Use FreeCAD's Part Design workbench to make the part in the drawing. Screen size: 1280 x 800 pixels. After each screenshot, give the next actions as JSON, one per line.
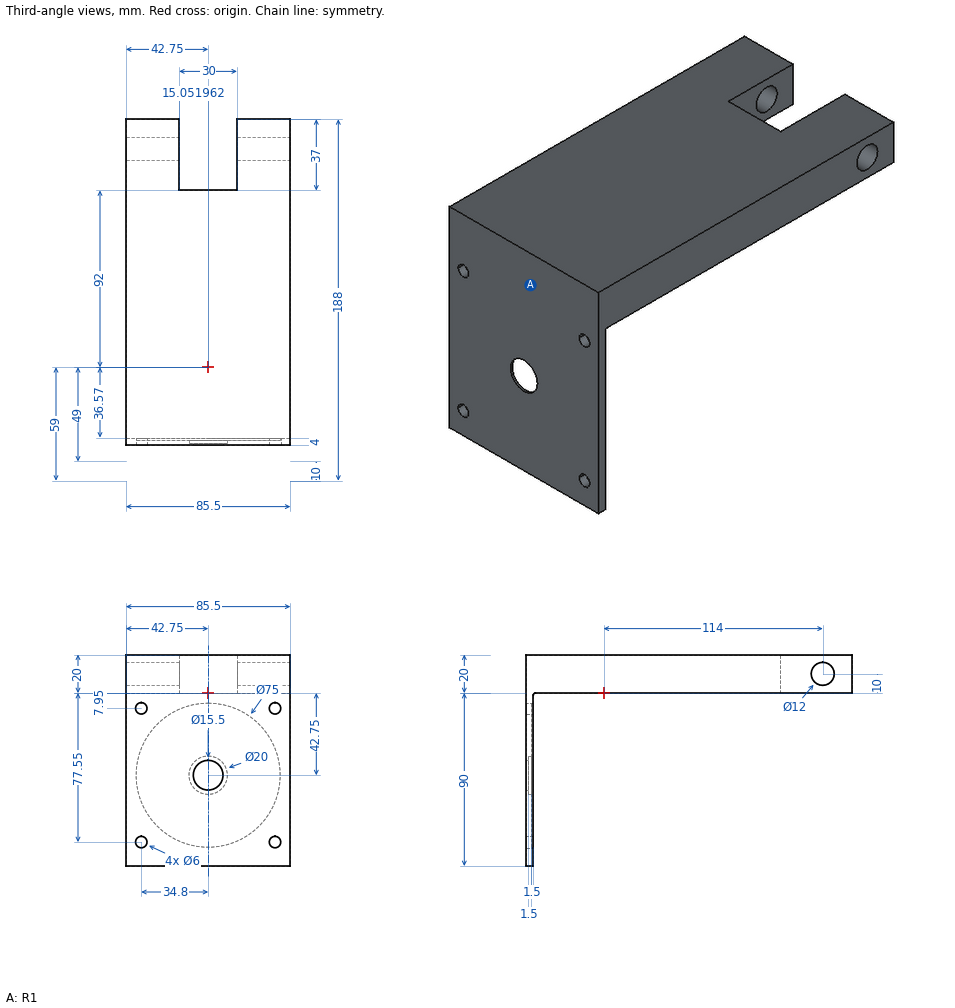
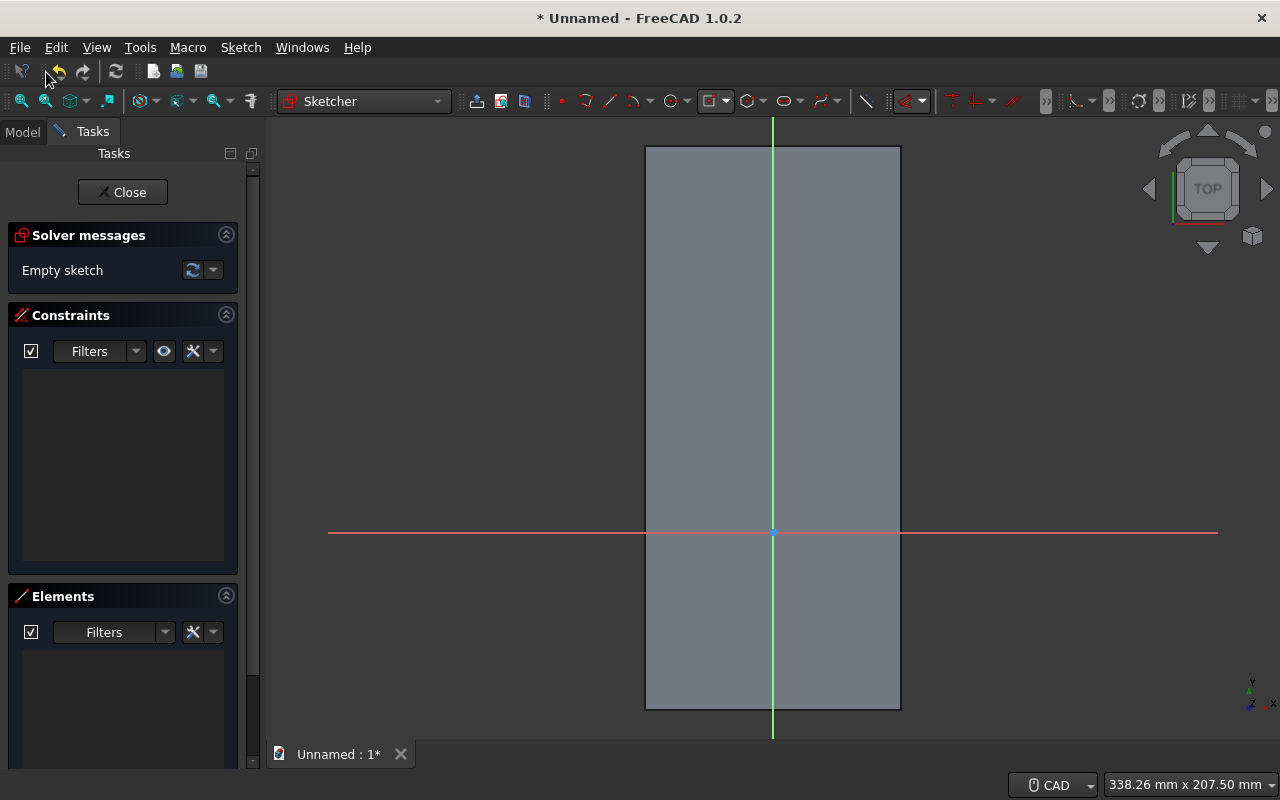
{"action": "scroll", "coordinate": [704, 428], "scroll_direction": "down", "scroll_amount": 5}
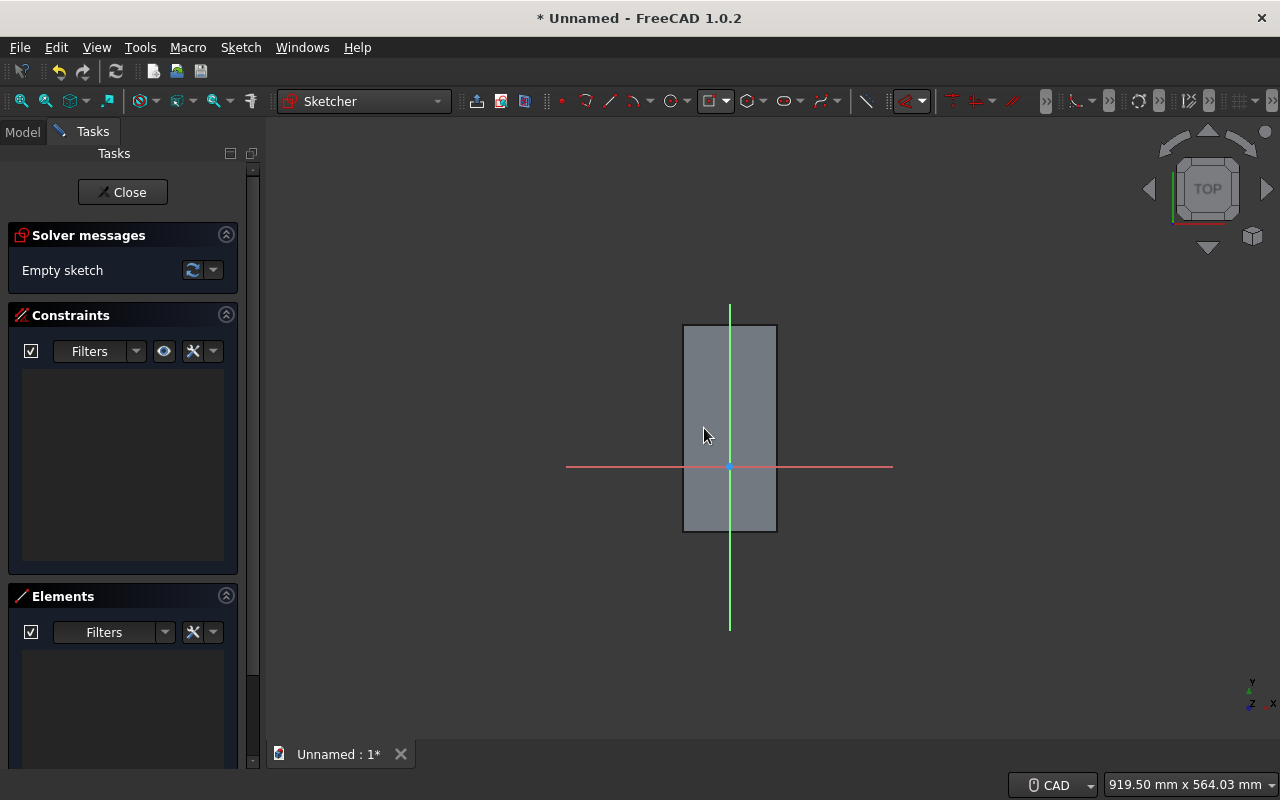
{"action": "scroll", "coordinate": [733, 335], "scroll_direction": "up", "scroll_amount": 11}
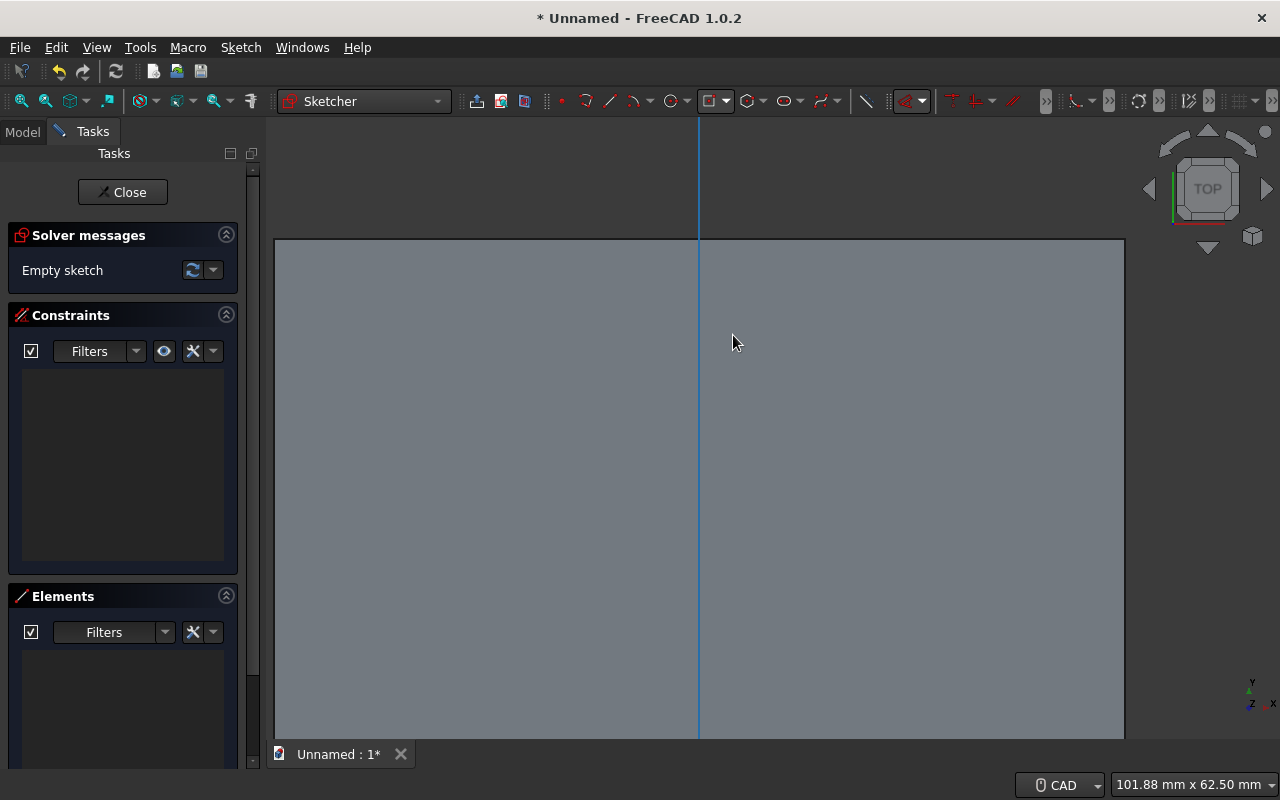
{"action": "key", "text": "g r"}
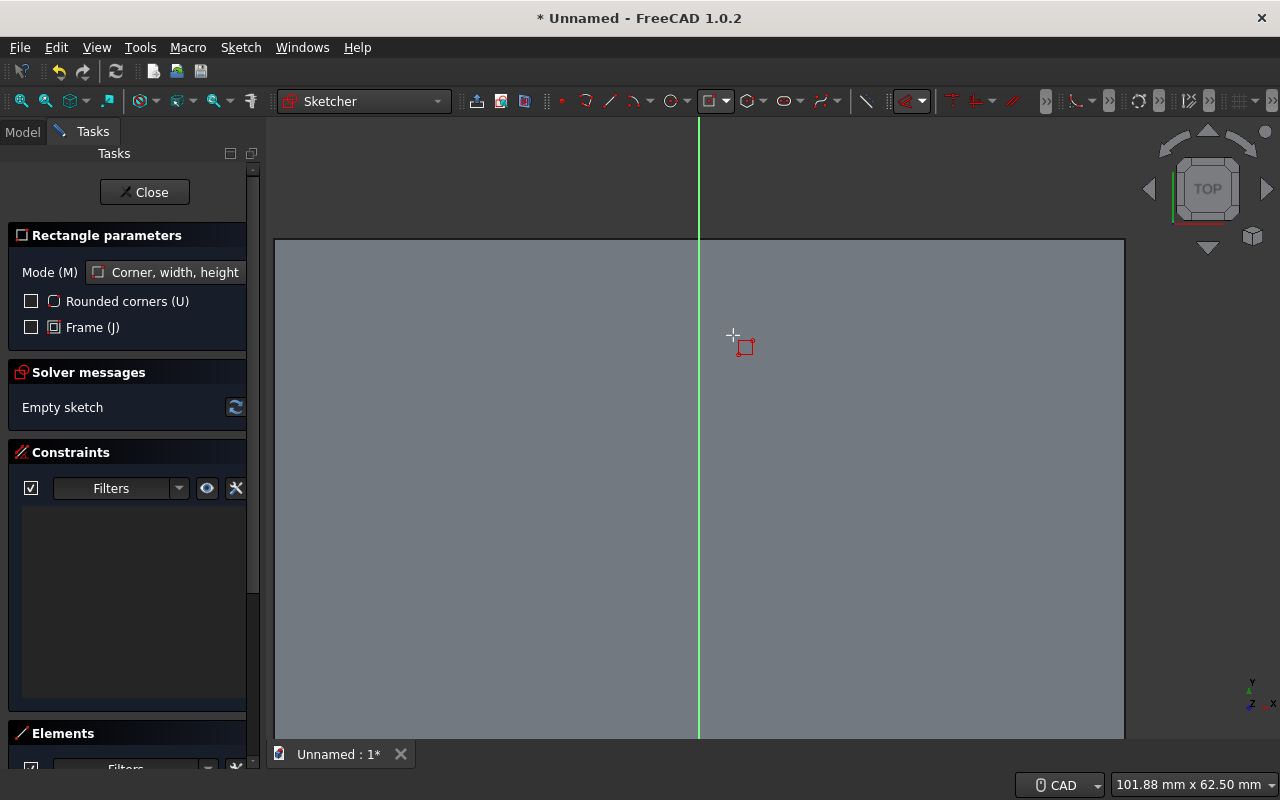
{"action": "left_click", "coordinate": [549, 239]}
{"action": "mouse_move", "coordinate": [848, 607]}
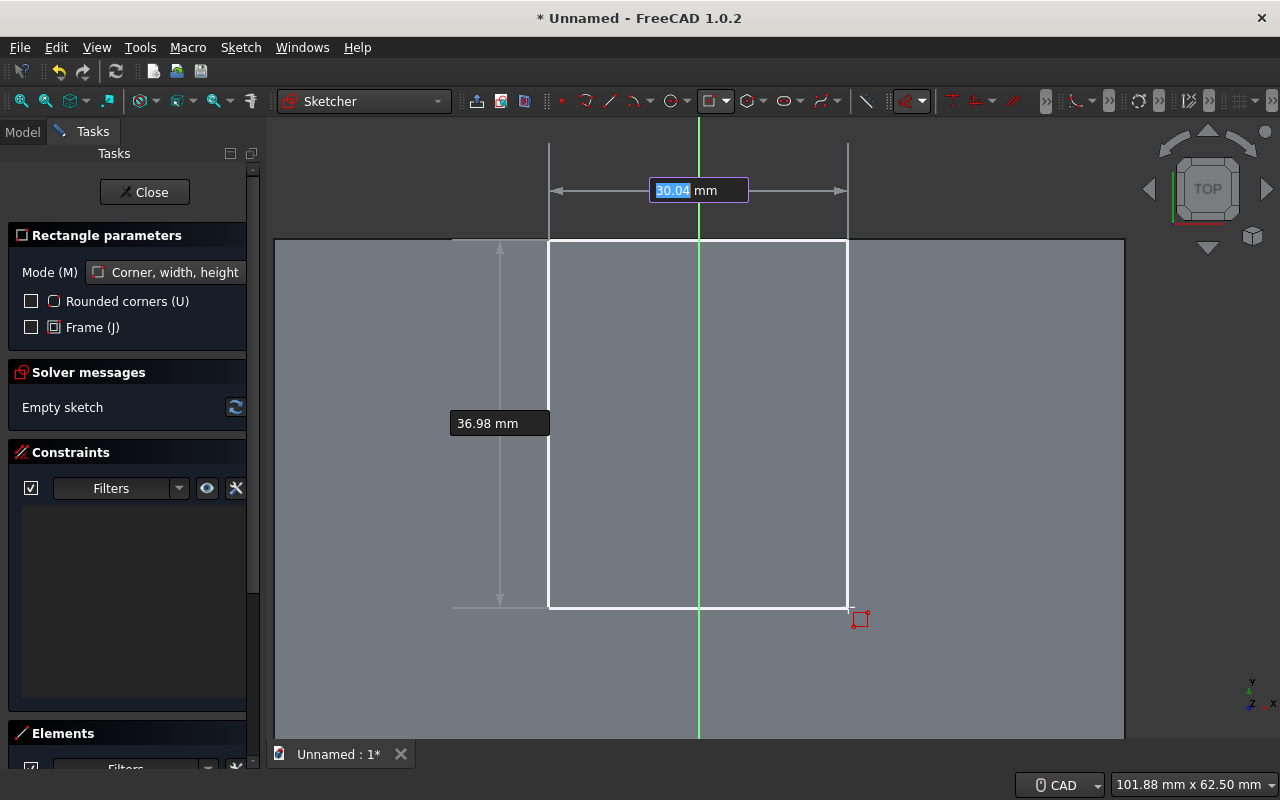
{"action": "type", "text": "30"}
{"action": "key", "text": "Tab"}
{"action": "type", "text": "37"}
{"action": "key", "text": "Return"}
{"action": "key", "text": "Escape"}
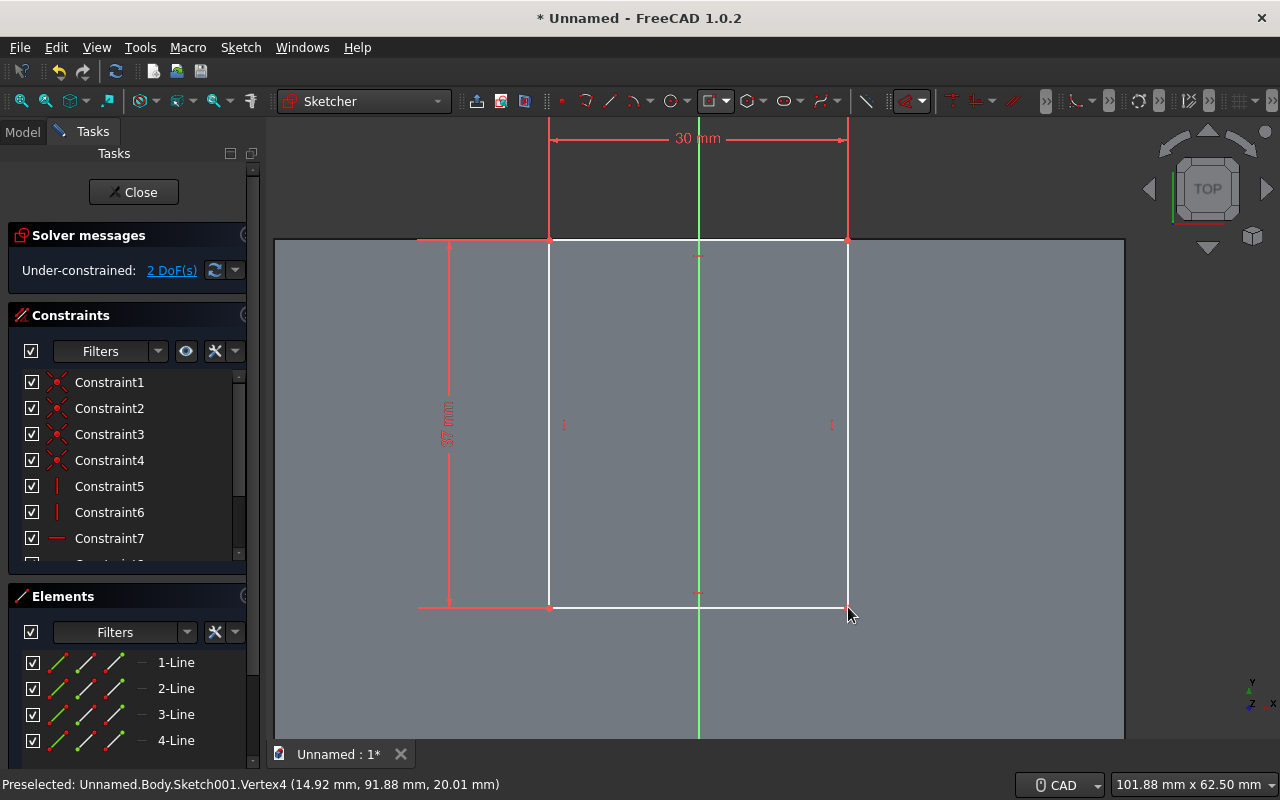
{"action": "left_click", "coordinate": [906, 102]}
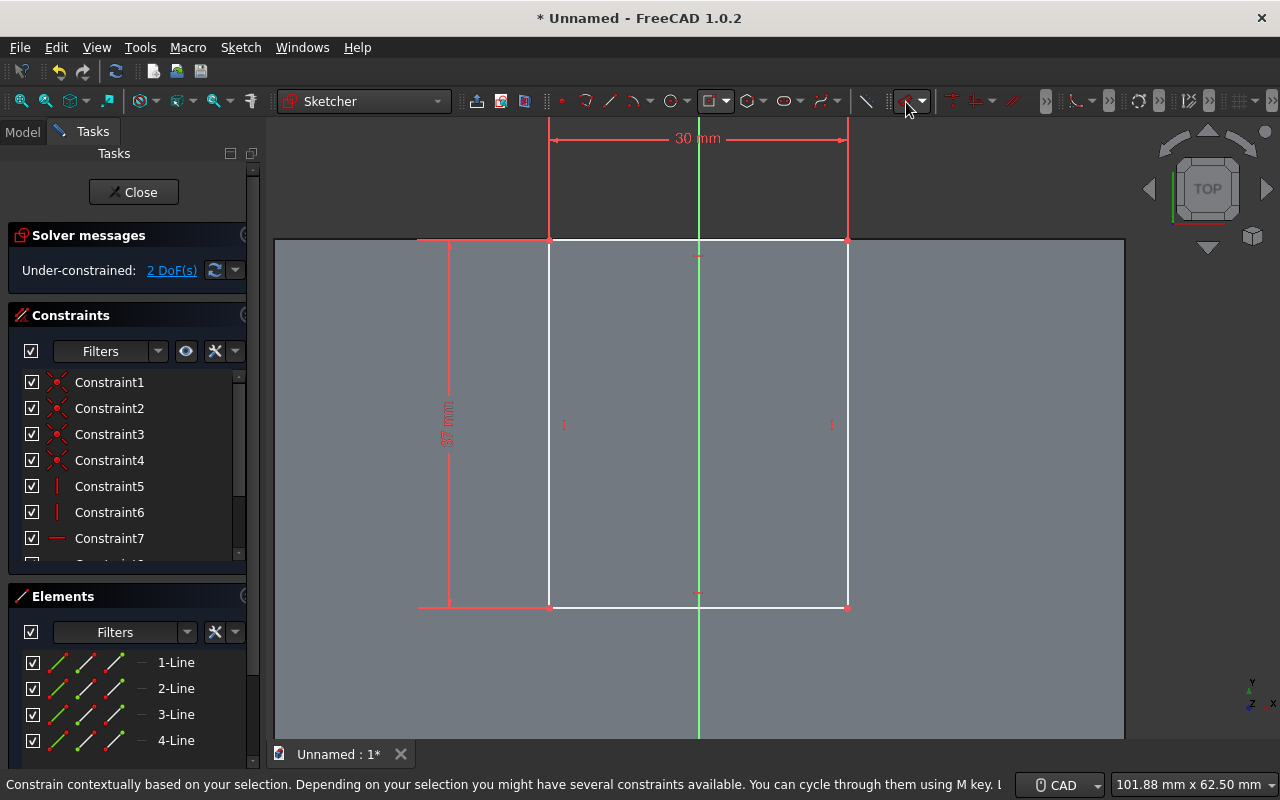
{"action": "left_click", "coordinate": [549, 608]}
{"action": "left_click", "coordinate": [515, 660]}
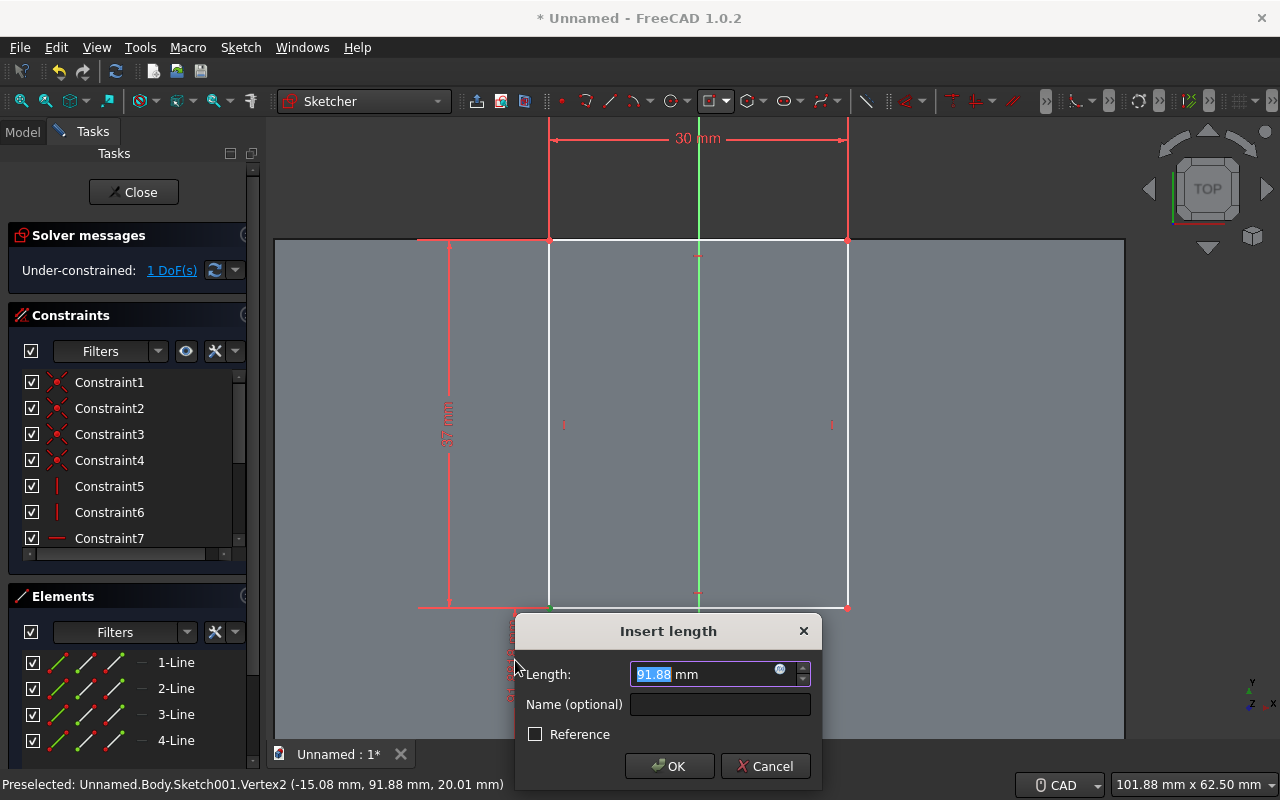
{"action": "type", "text": "92"}
{"action": "key", "text": "Return"}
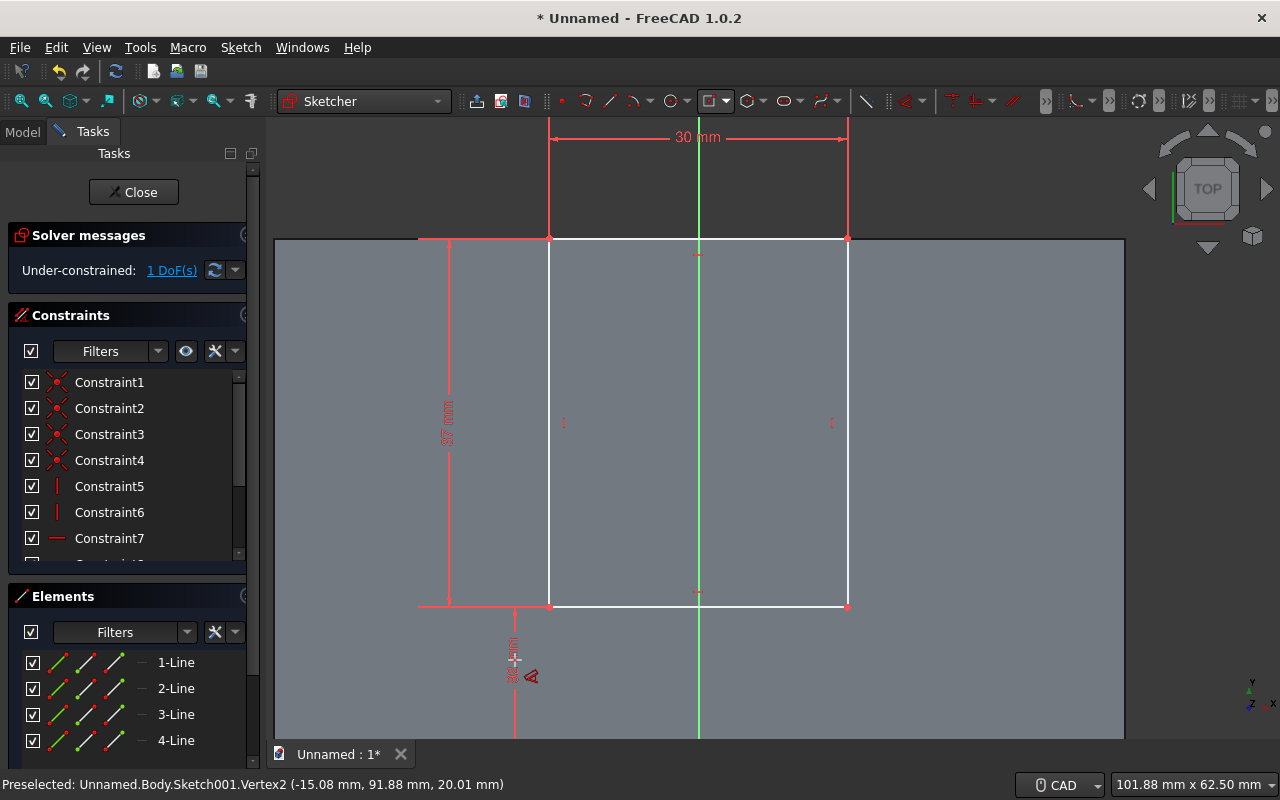
{"action": "left_click", "coordinate": [549, 239]}
{"action": "left_click", "coordinate": [624, 205]}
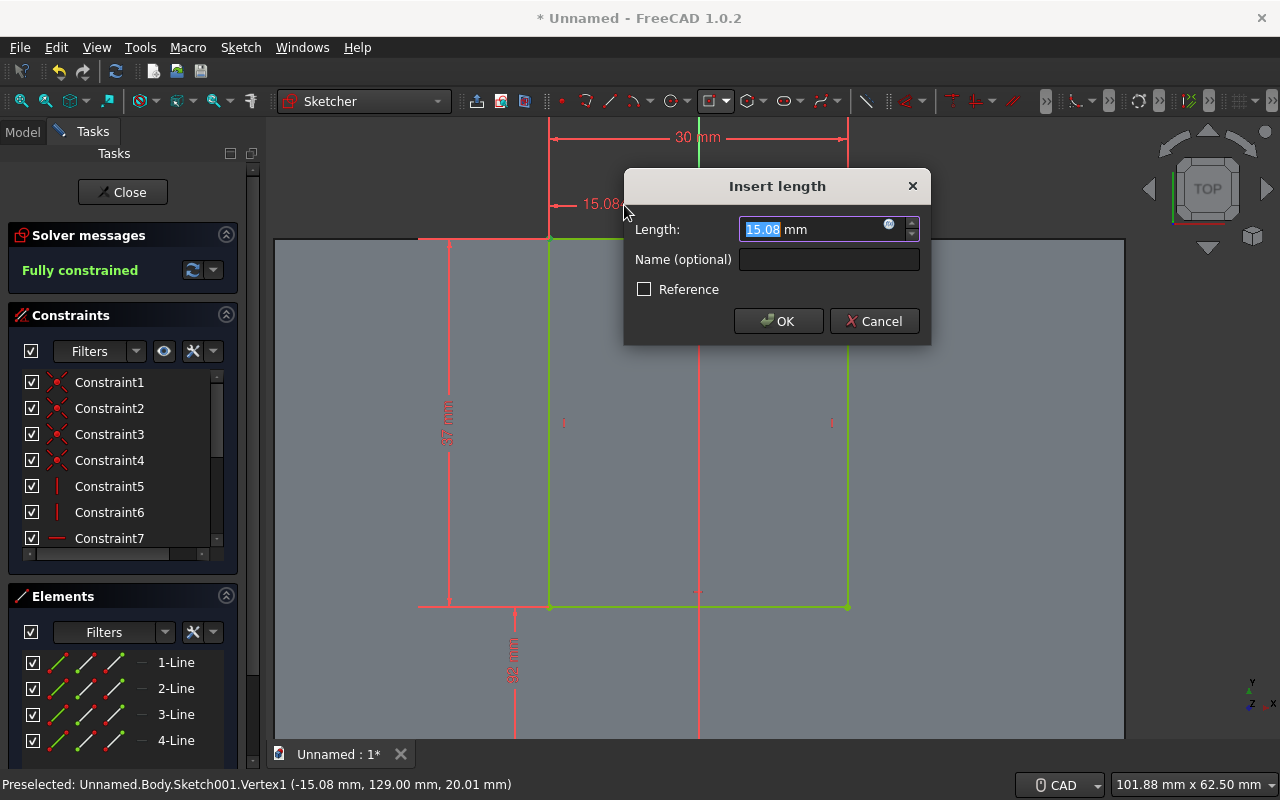
{"action": "type", "text": "15.051962"}
{"action": "key", "text": "Return"}
{"action": "key", "text": "Escape"}